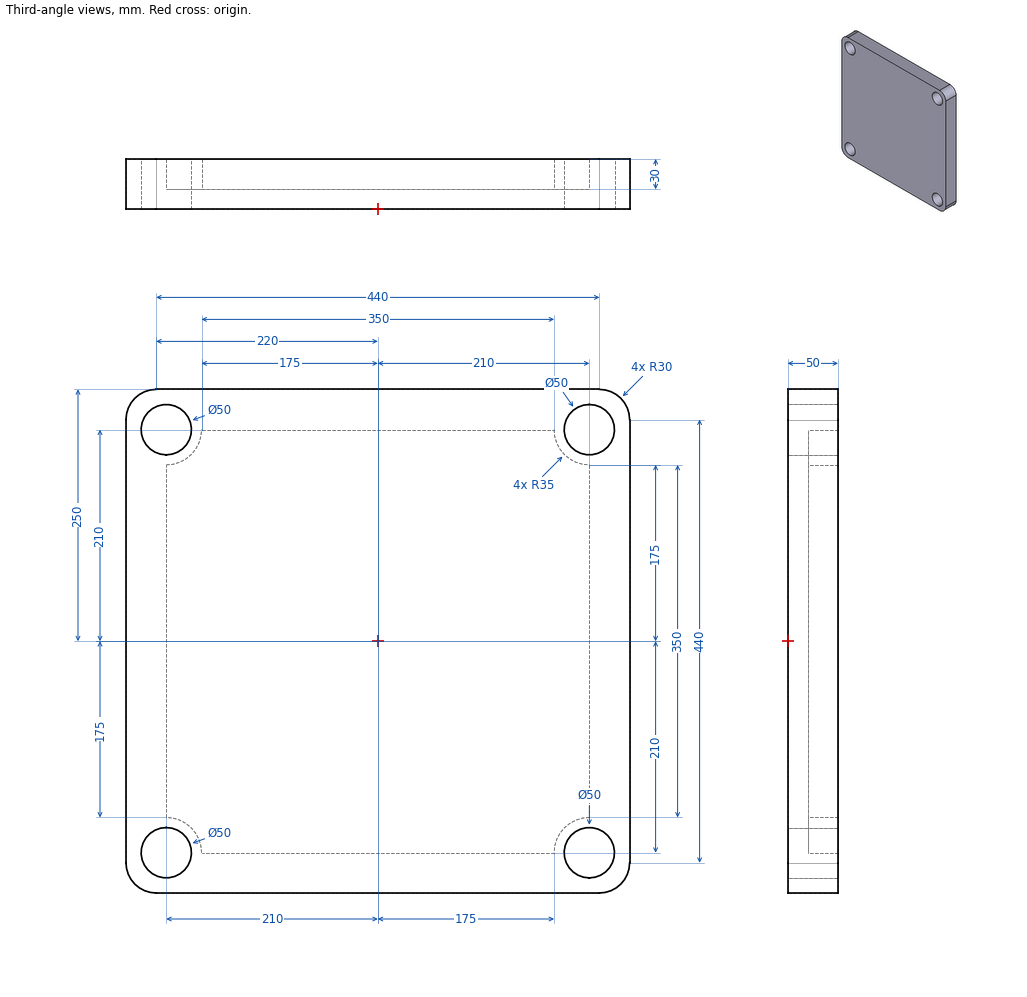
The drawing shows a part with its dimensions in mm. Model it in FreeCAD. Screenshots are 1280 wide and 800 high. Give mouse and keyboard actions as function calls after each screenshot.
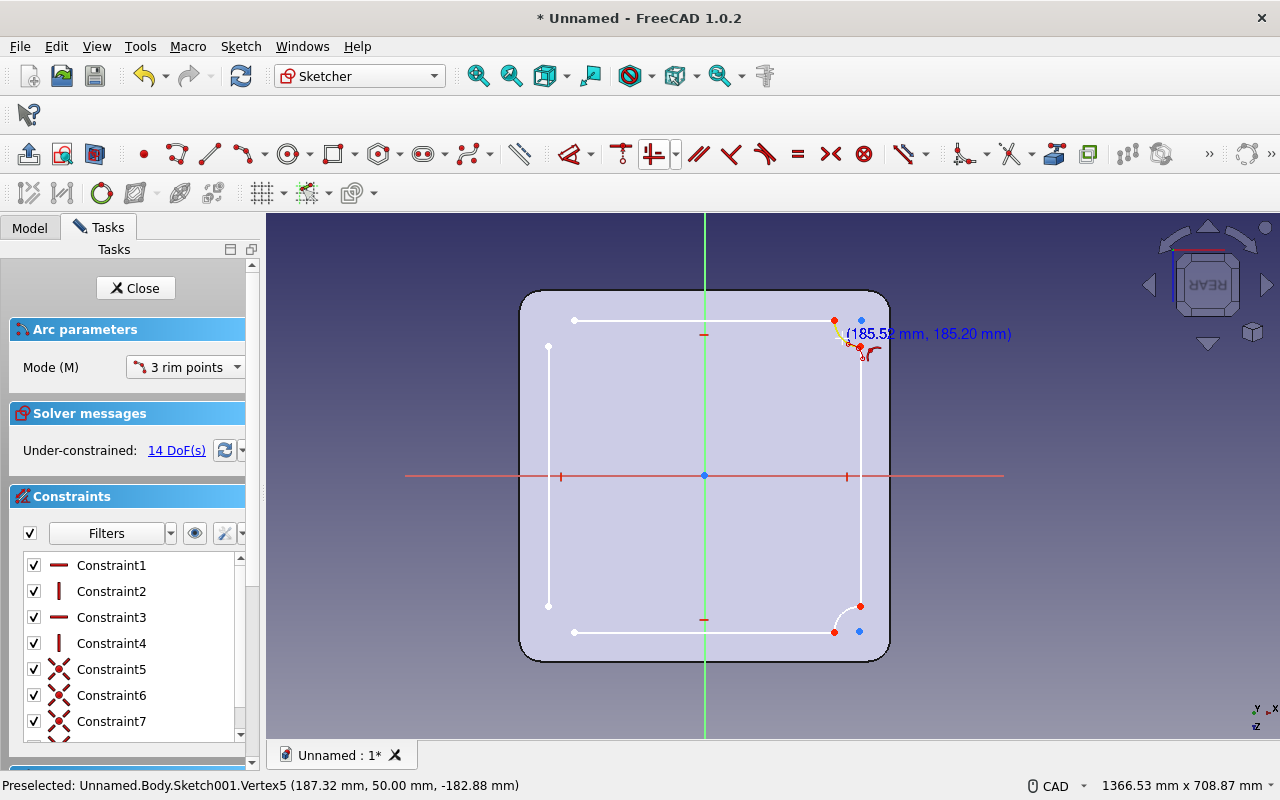
click(575, 321)
click(549, 347)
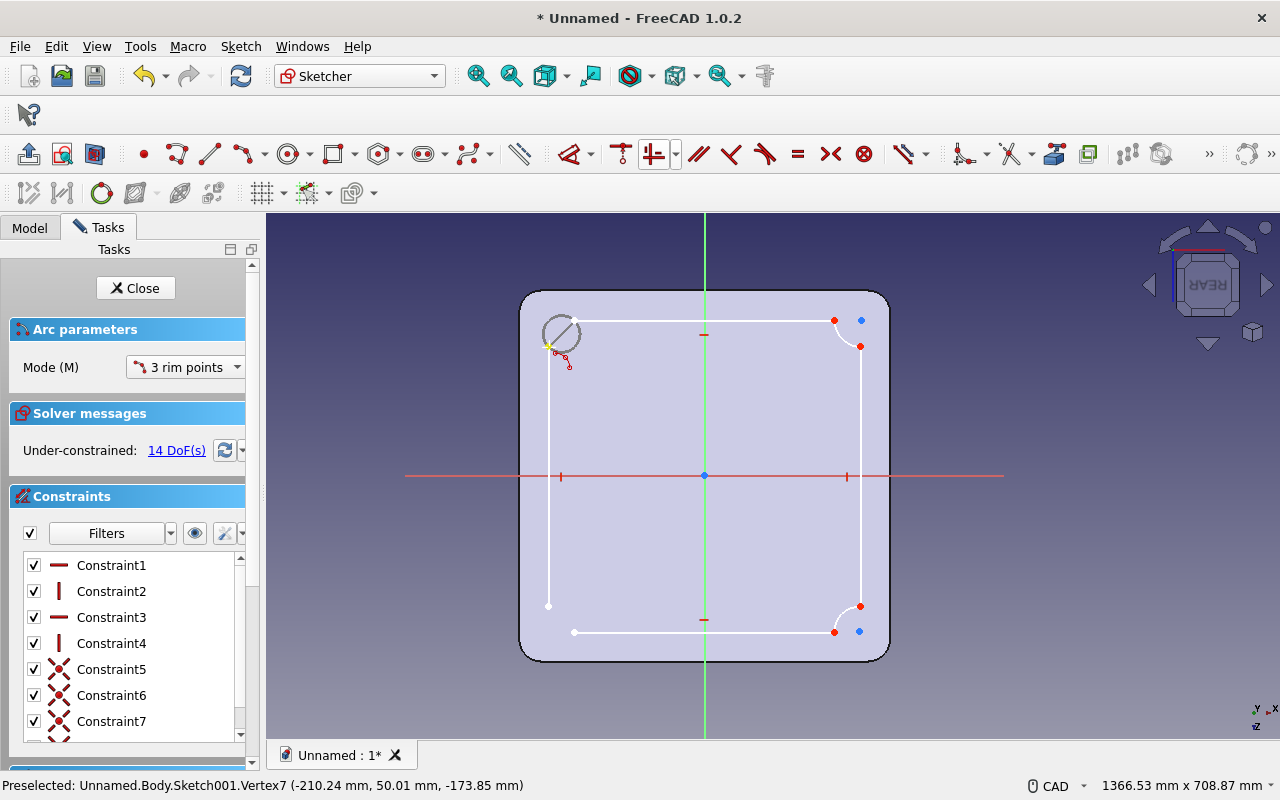
scroll(567, 339, up, 4)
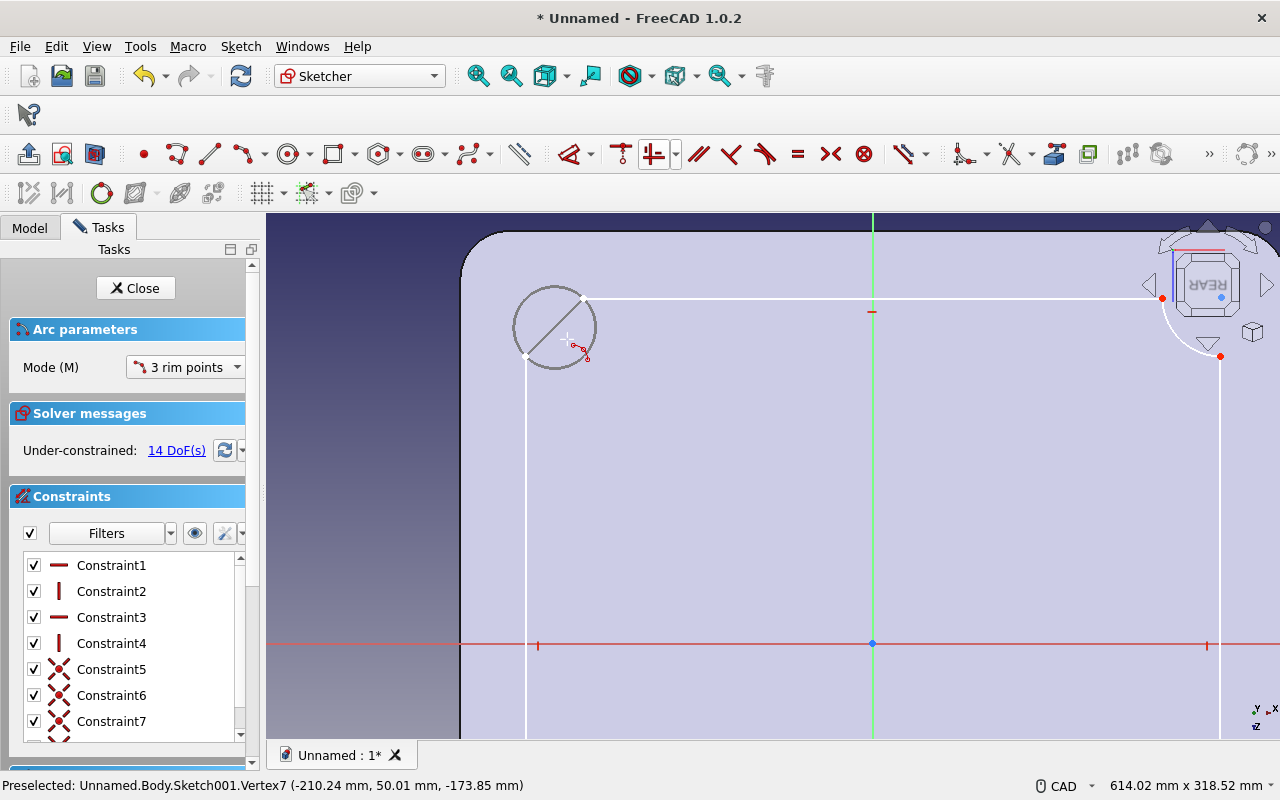
click(567, 338)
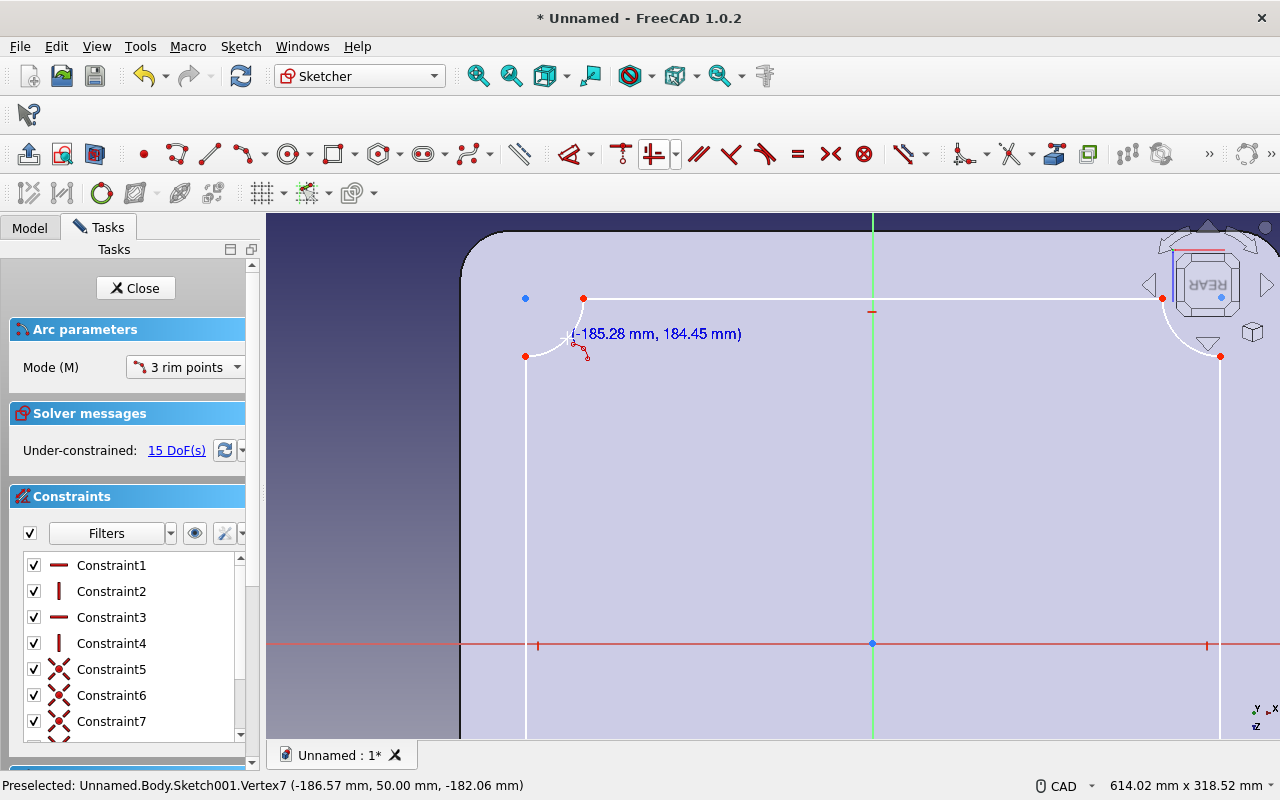
scroll(567, 339, down, 4)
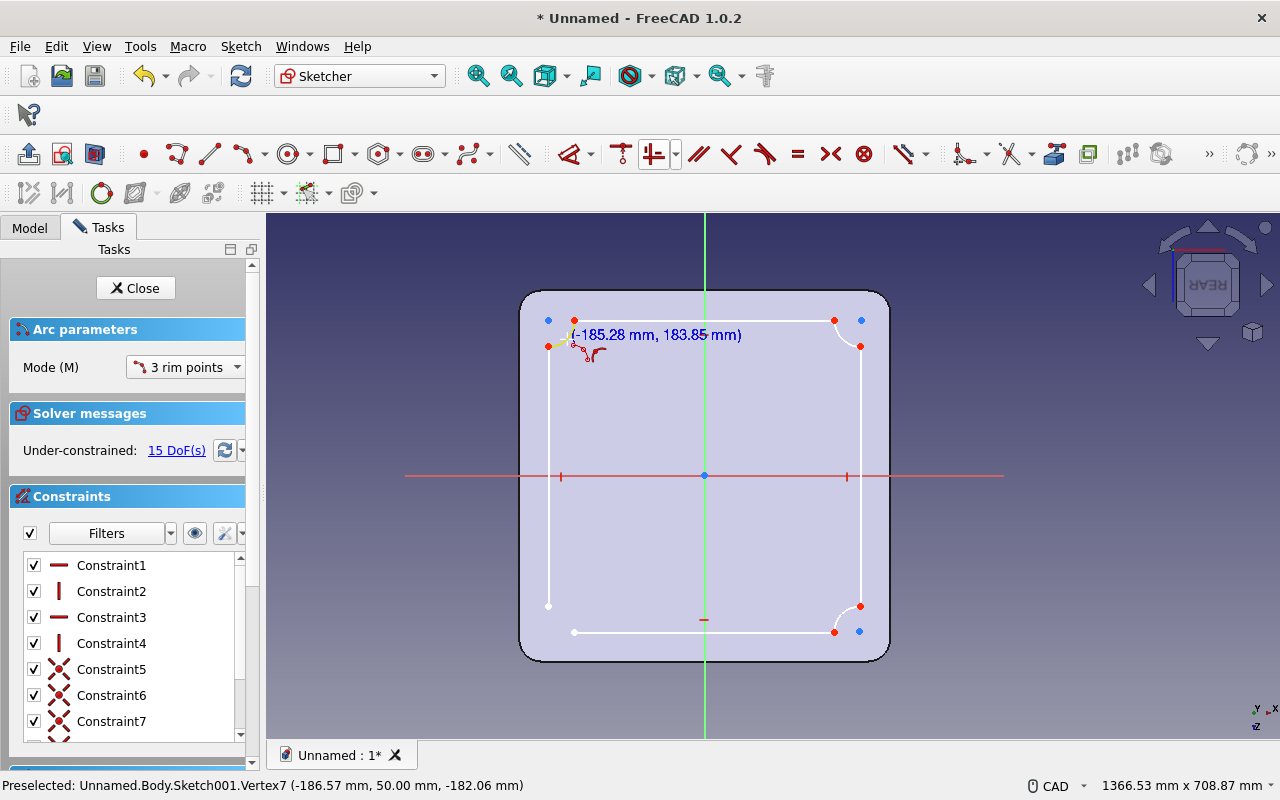
click(549, 607)
click(575, 633)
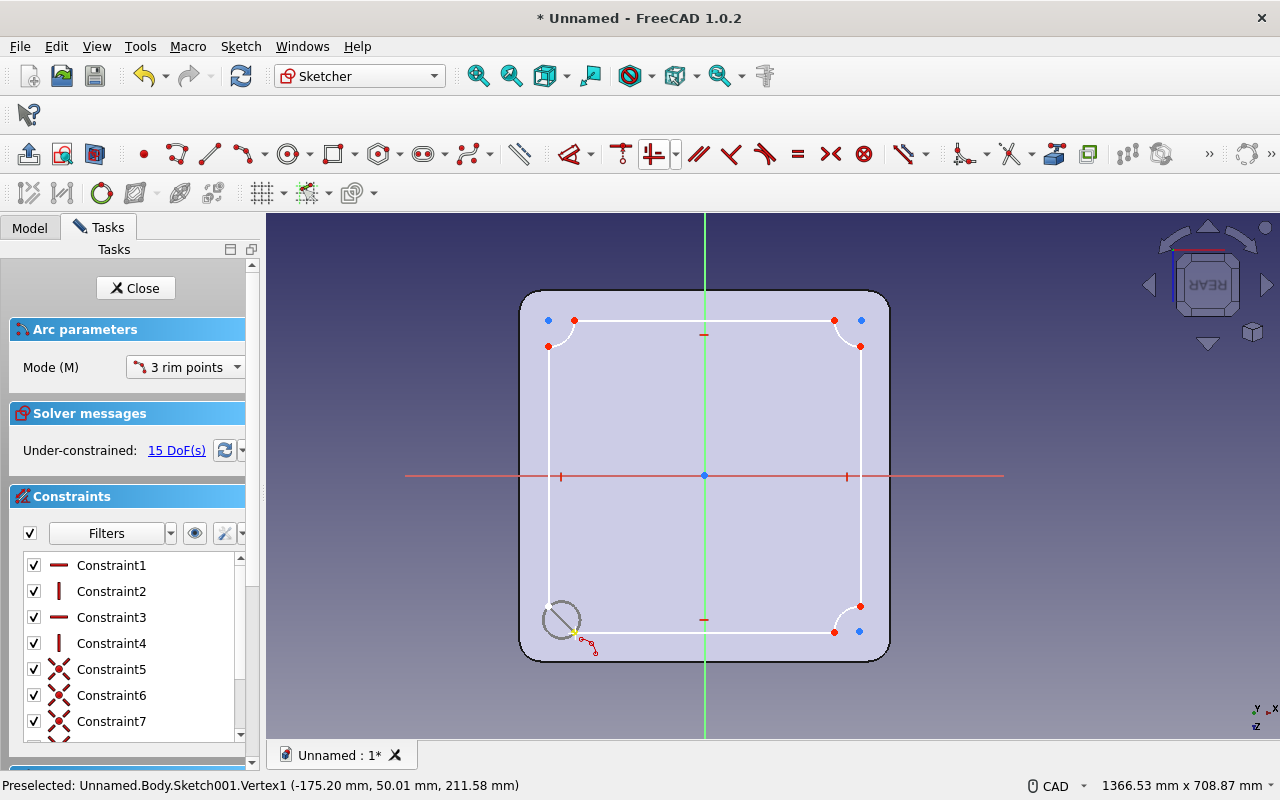
scroll(567, 613, up, 4)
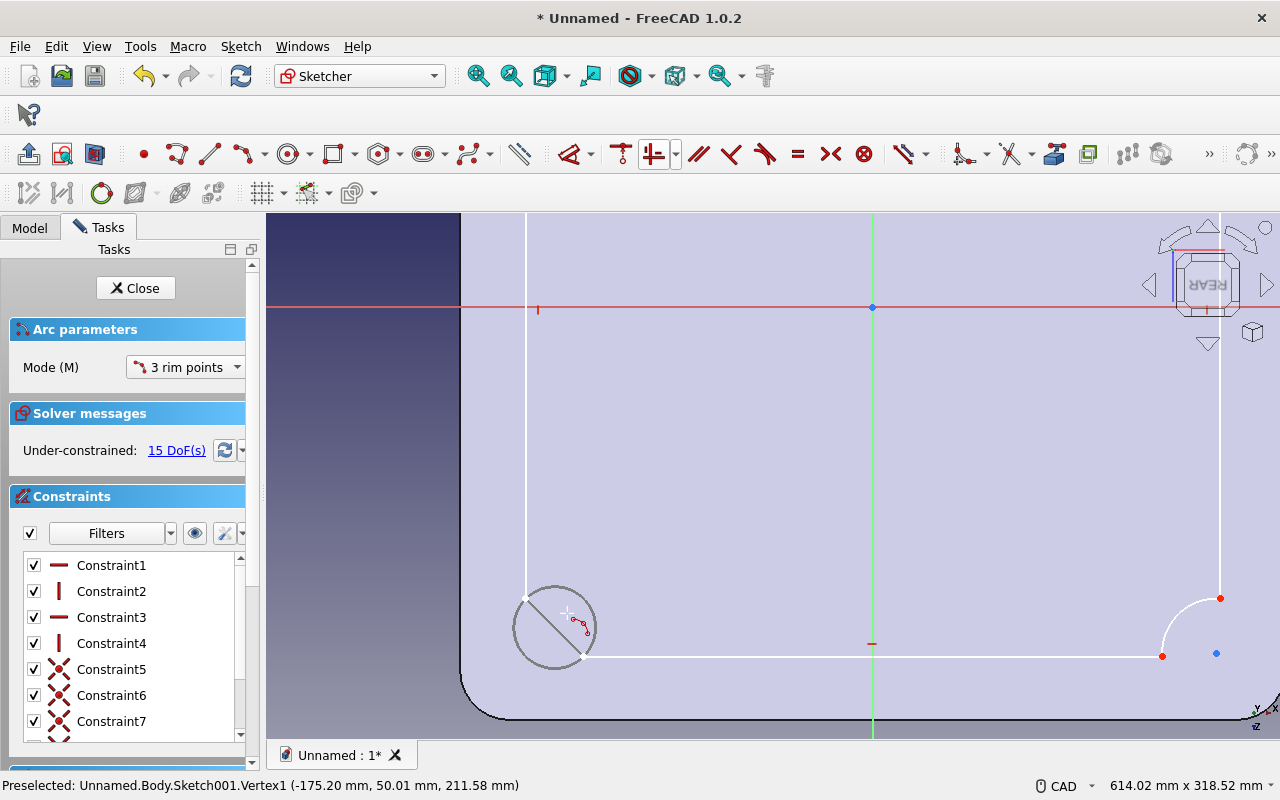
click(567, 613)
key(Escape)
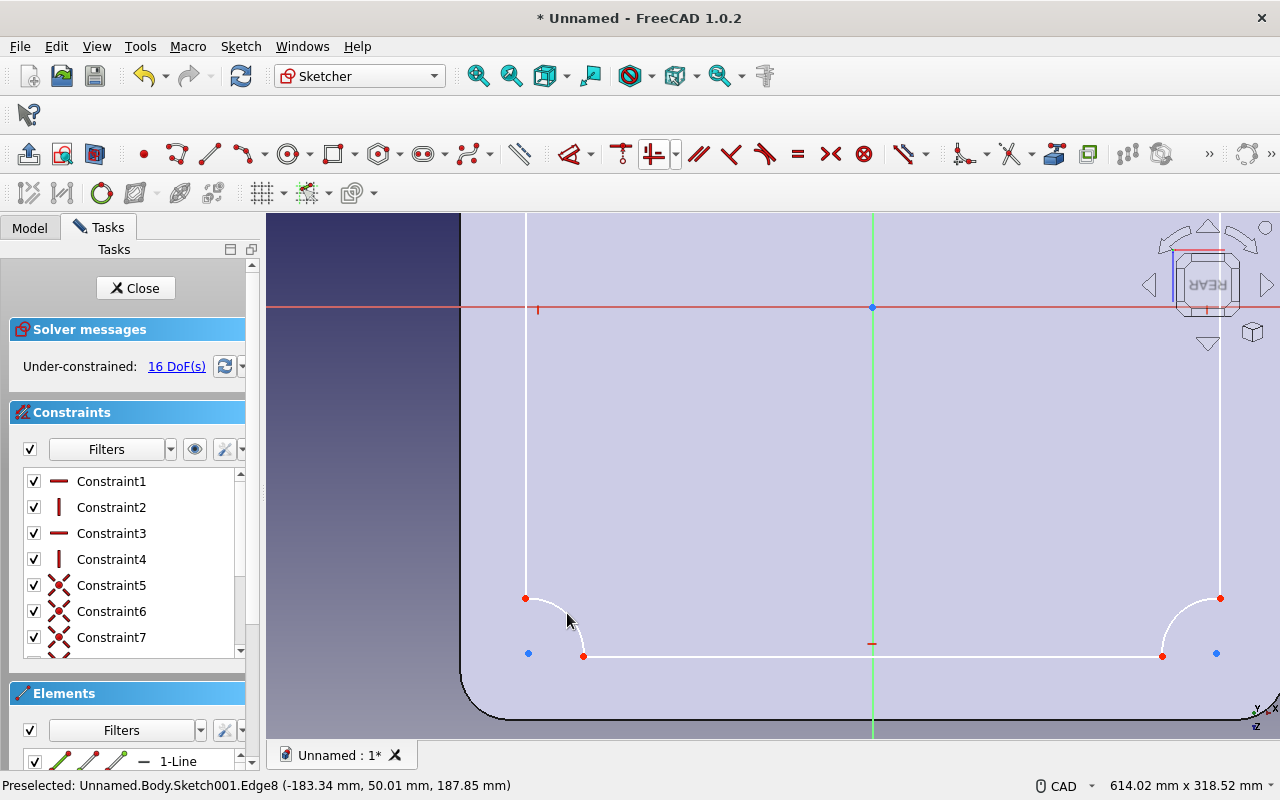
scroll(567, 614, down, 4)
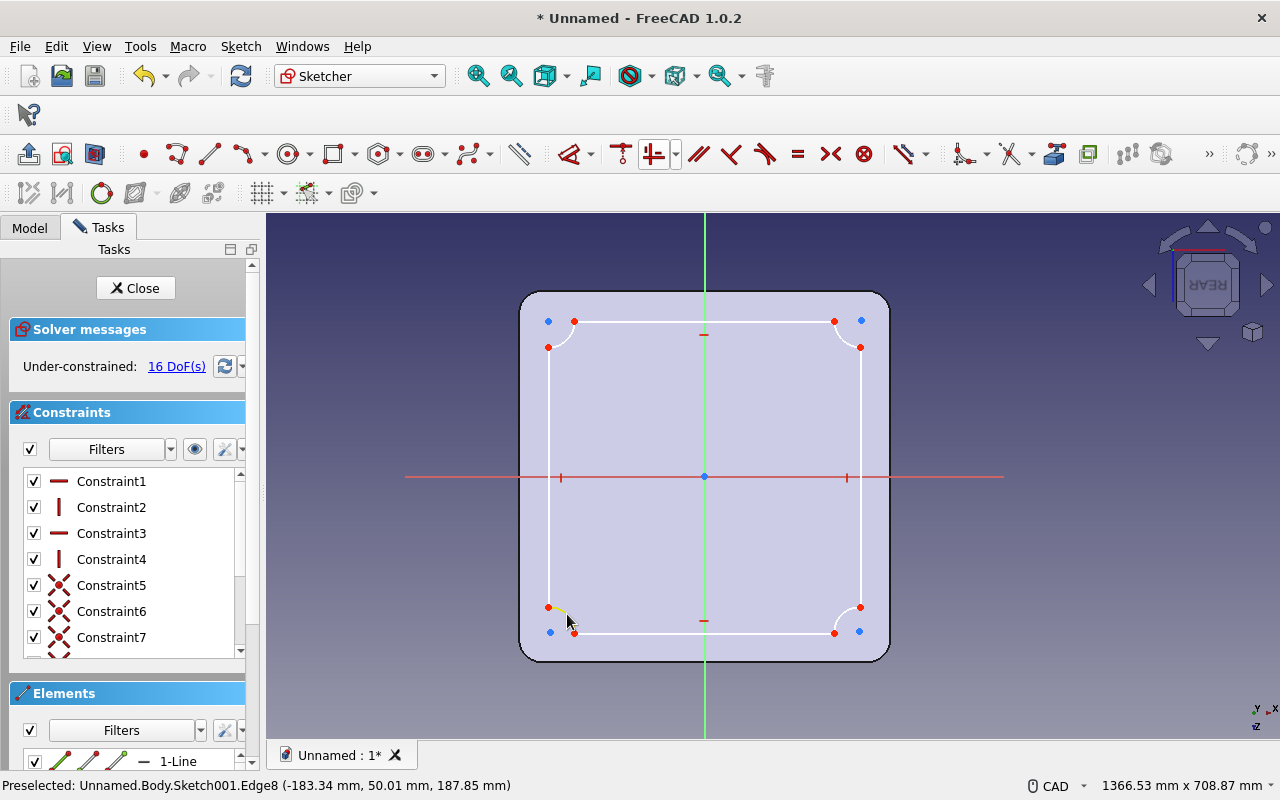
click(849, 610)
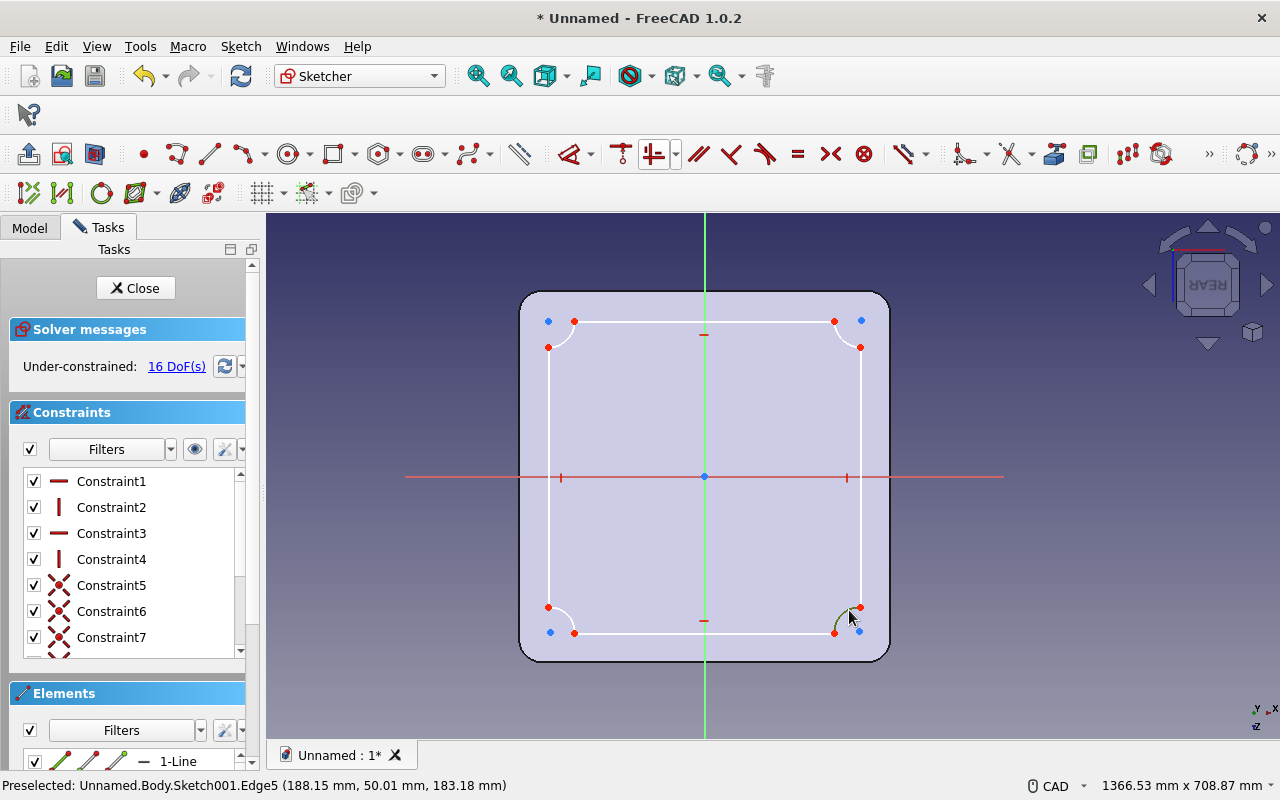
click(838, 333)